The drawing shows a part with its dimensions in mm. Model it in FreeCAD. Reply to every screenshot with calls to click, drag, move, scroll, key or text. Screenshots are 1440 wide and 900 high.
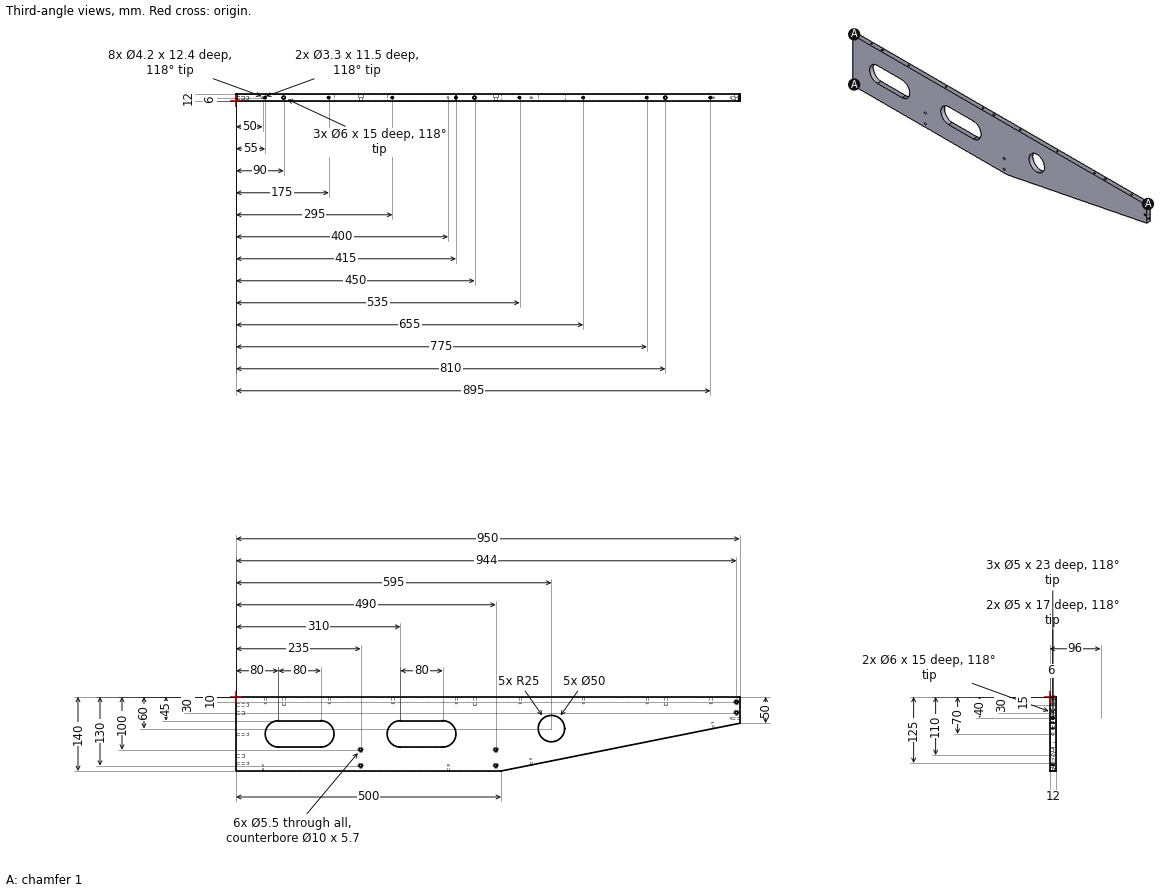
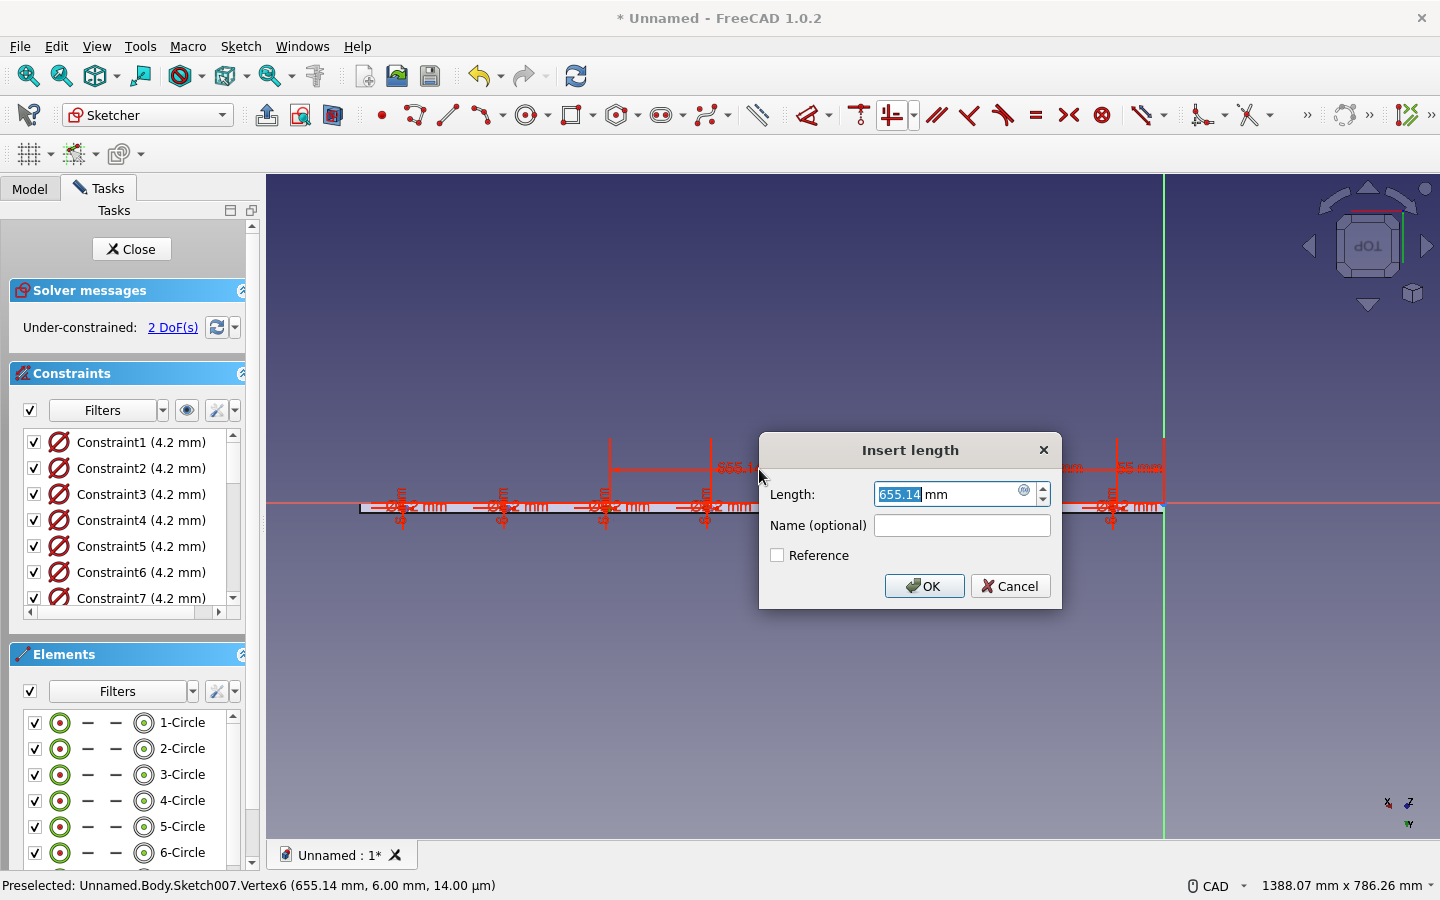
text(655)
key(Return)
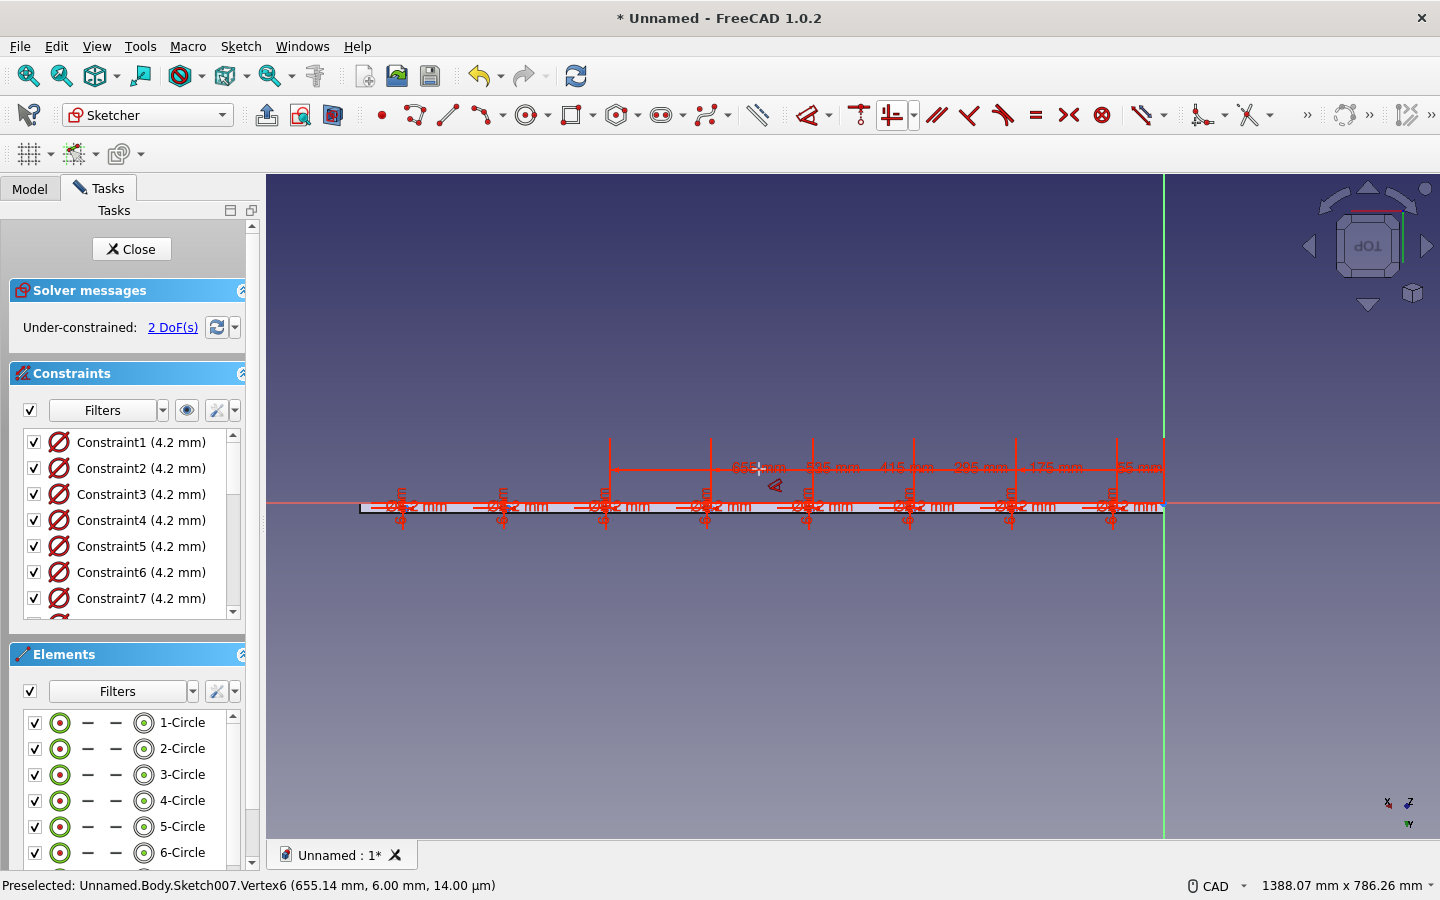
click(508, 508)
click(685, 469)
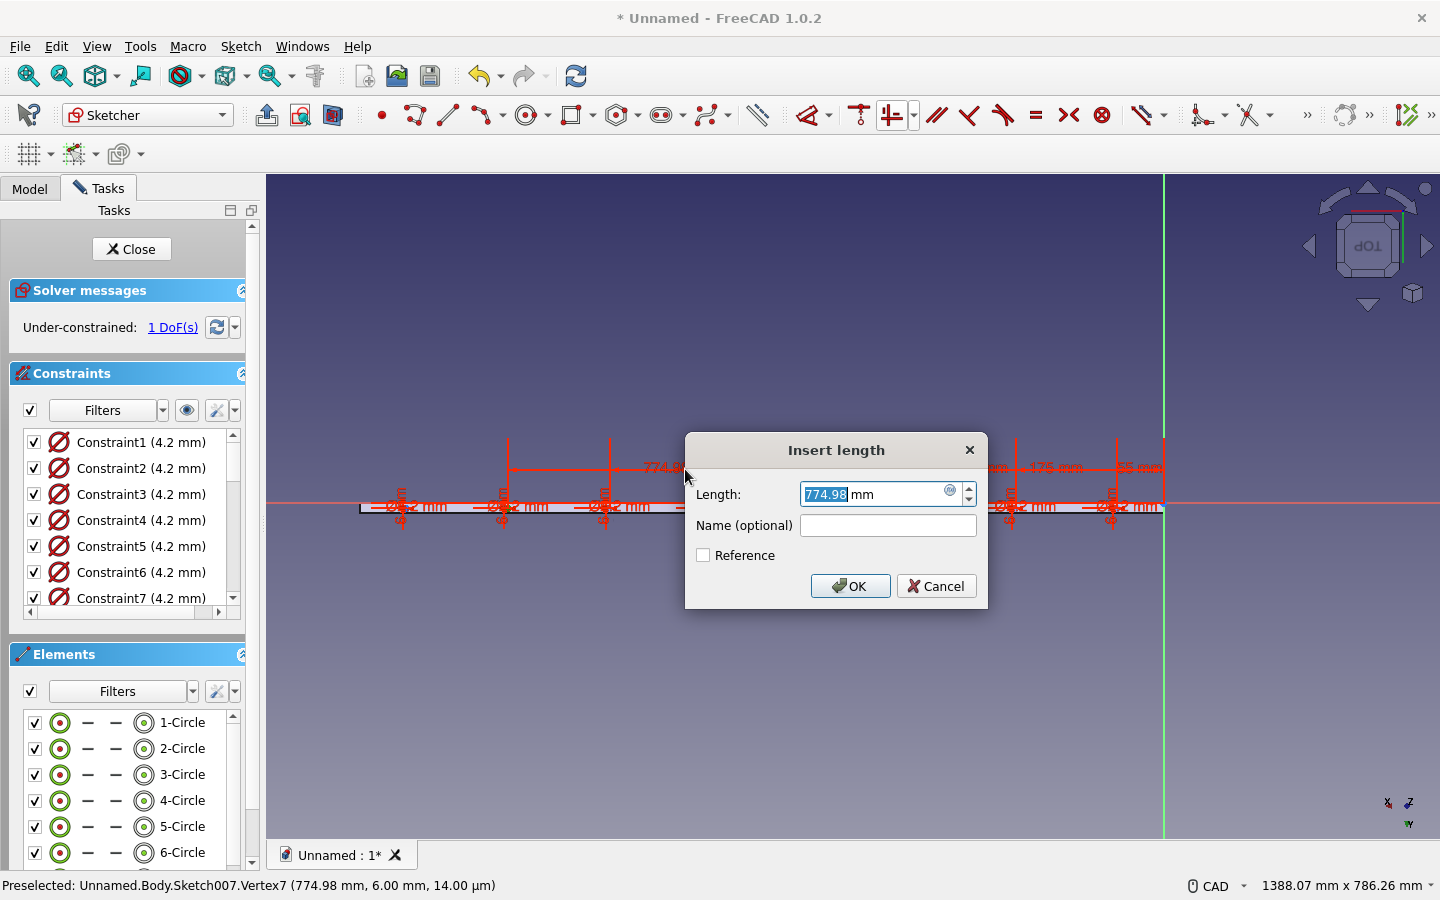
text(775)
key(Return)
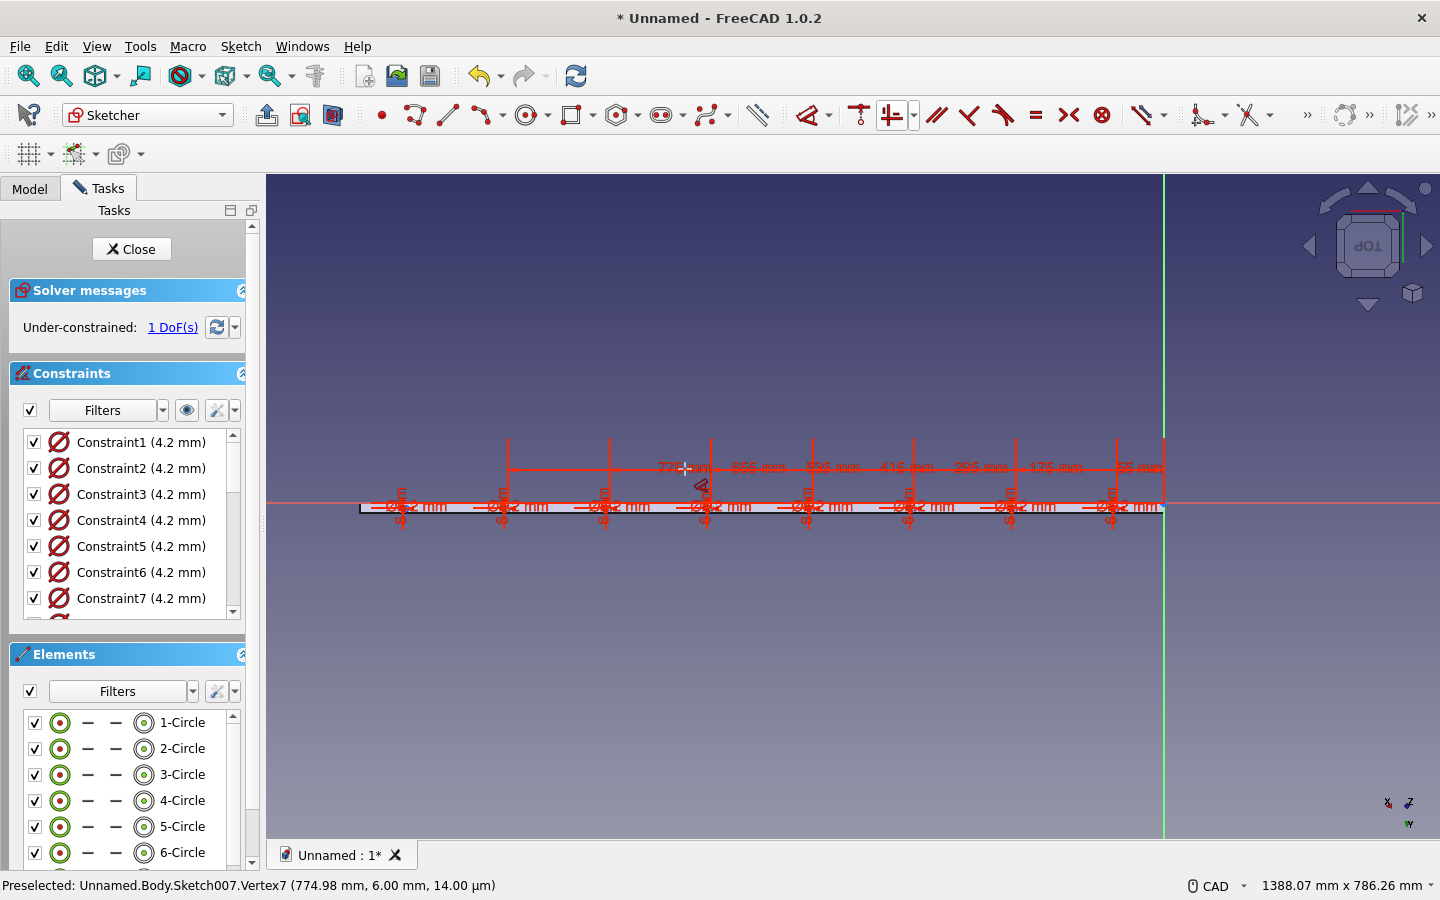
click(407, 508)
click(611, 469)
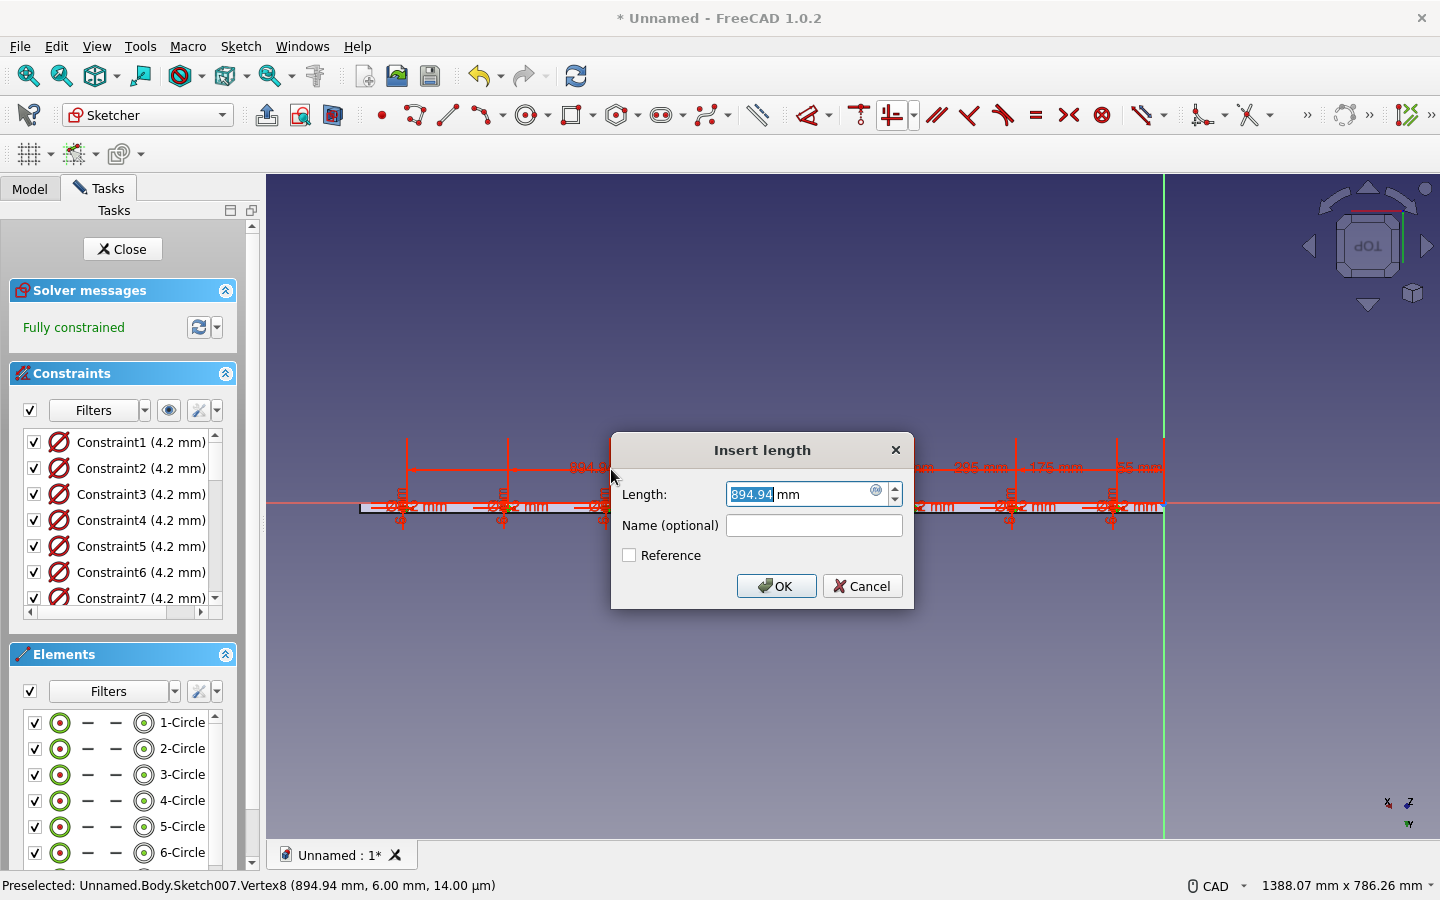
text(895)
key(Return)
key(Escape)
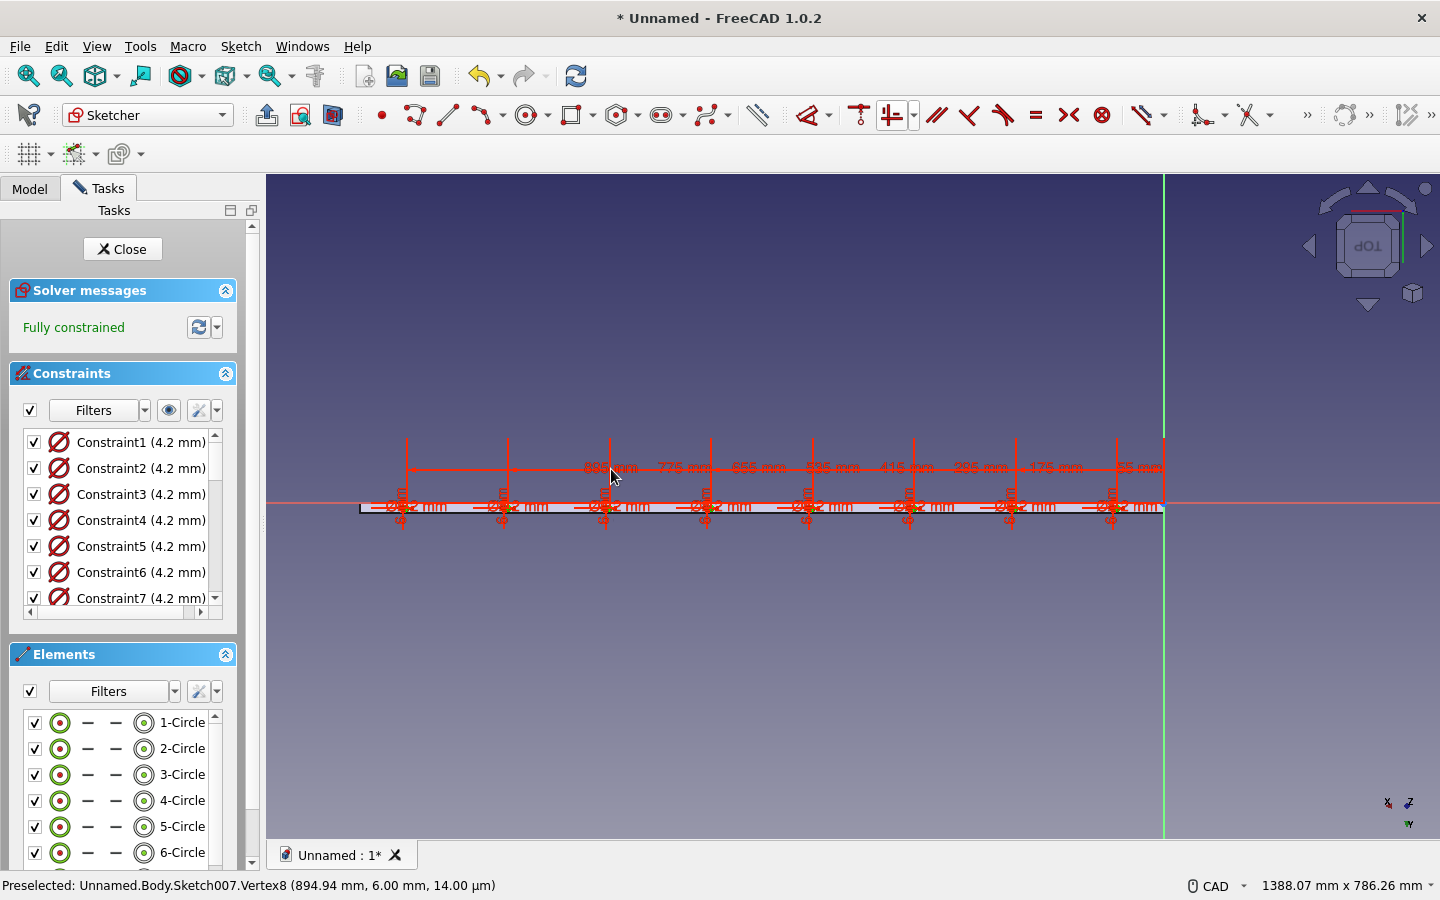
click(123, 249)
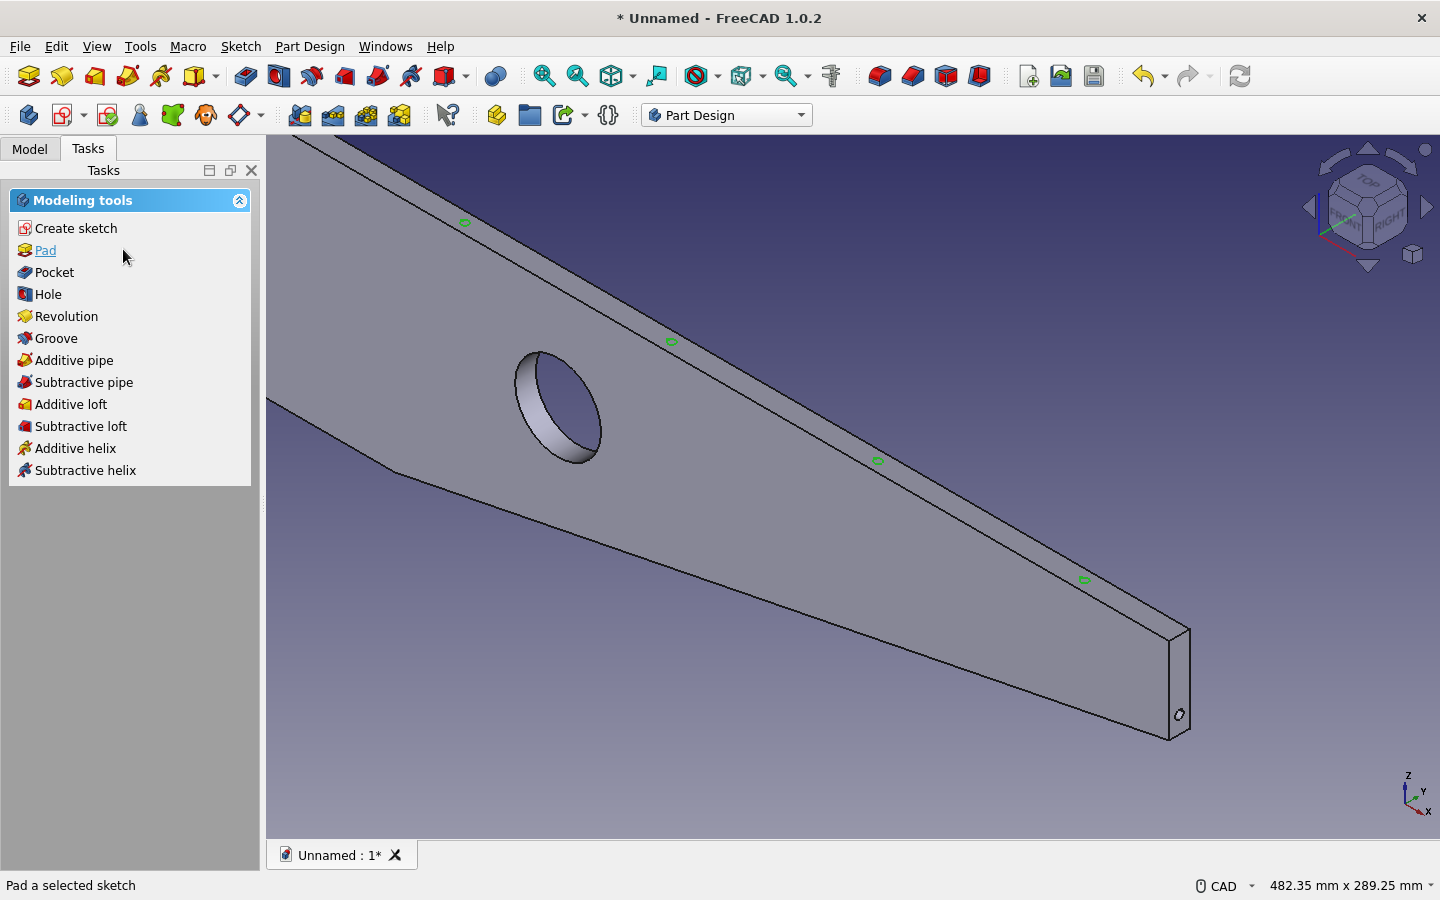
click(279, 76)